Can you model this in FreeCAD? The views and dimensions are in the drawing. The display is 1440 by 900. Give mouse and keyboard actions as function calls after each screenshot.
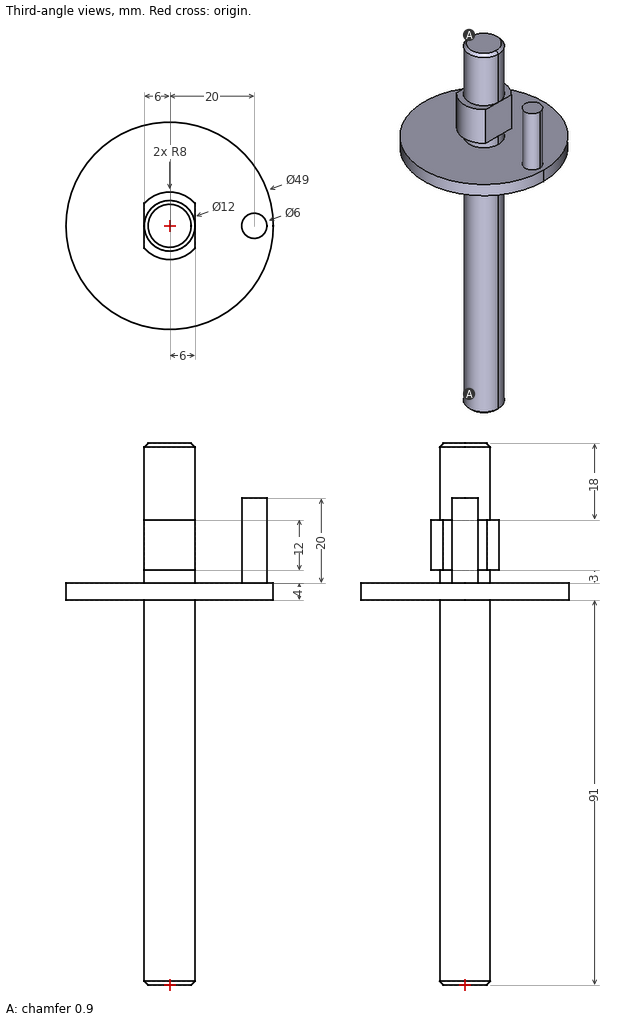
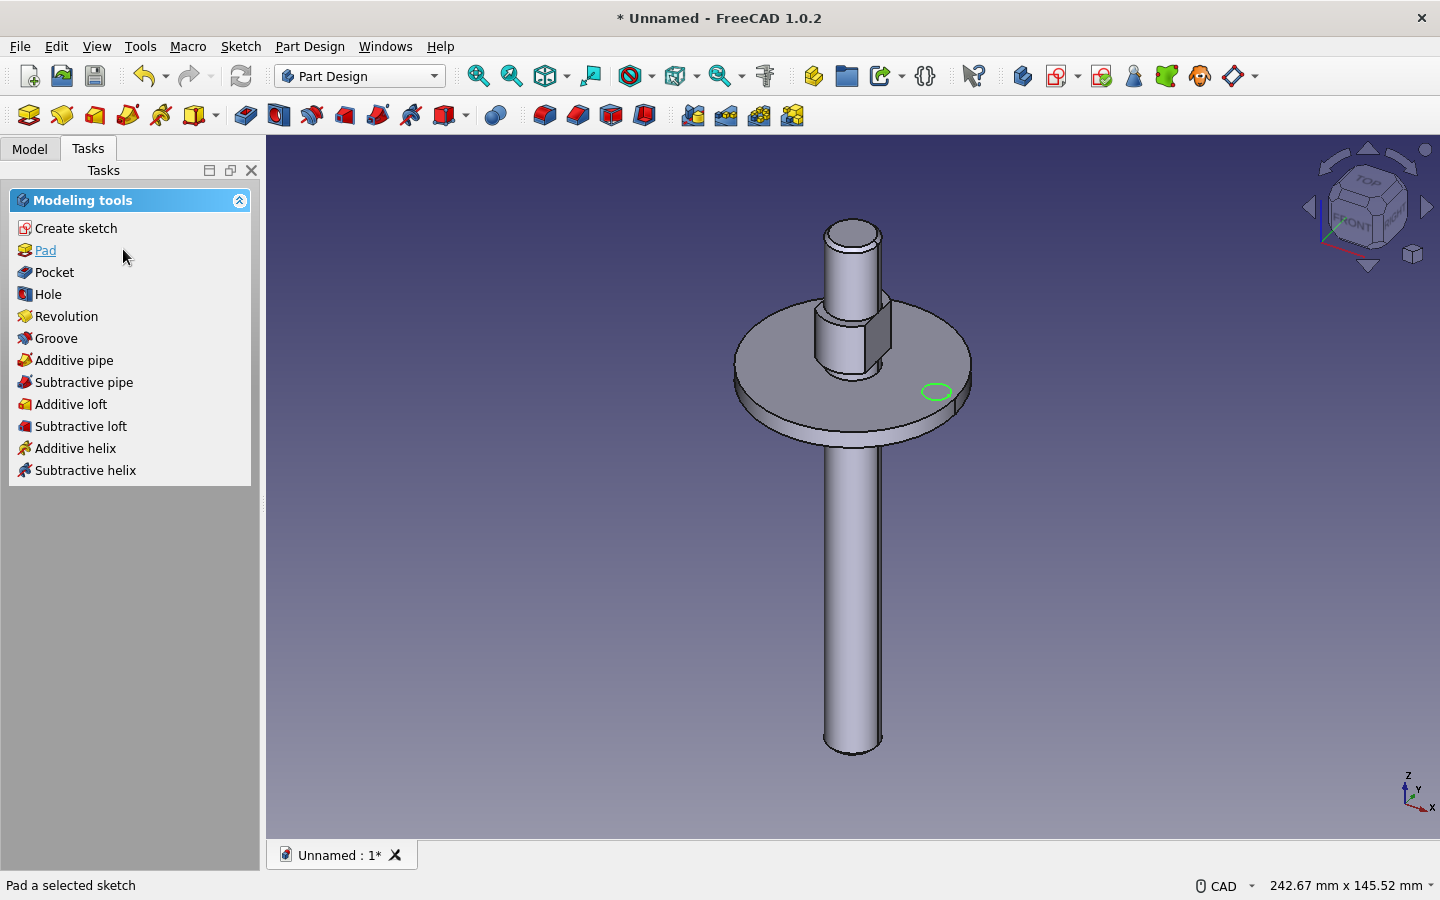
click(29, 116)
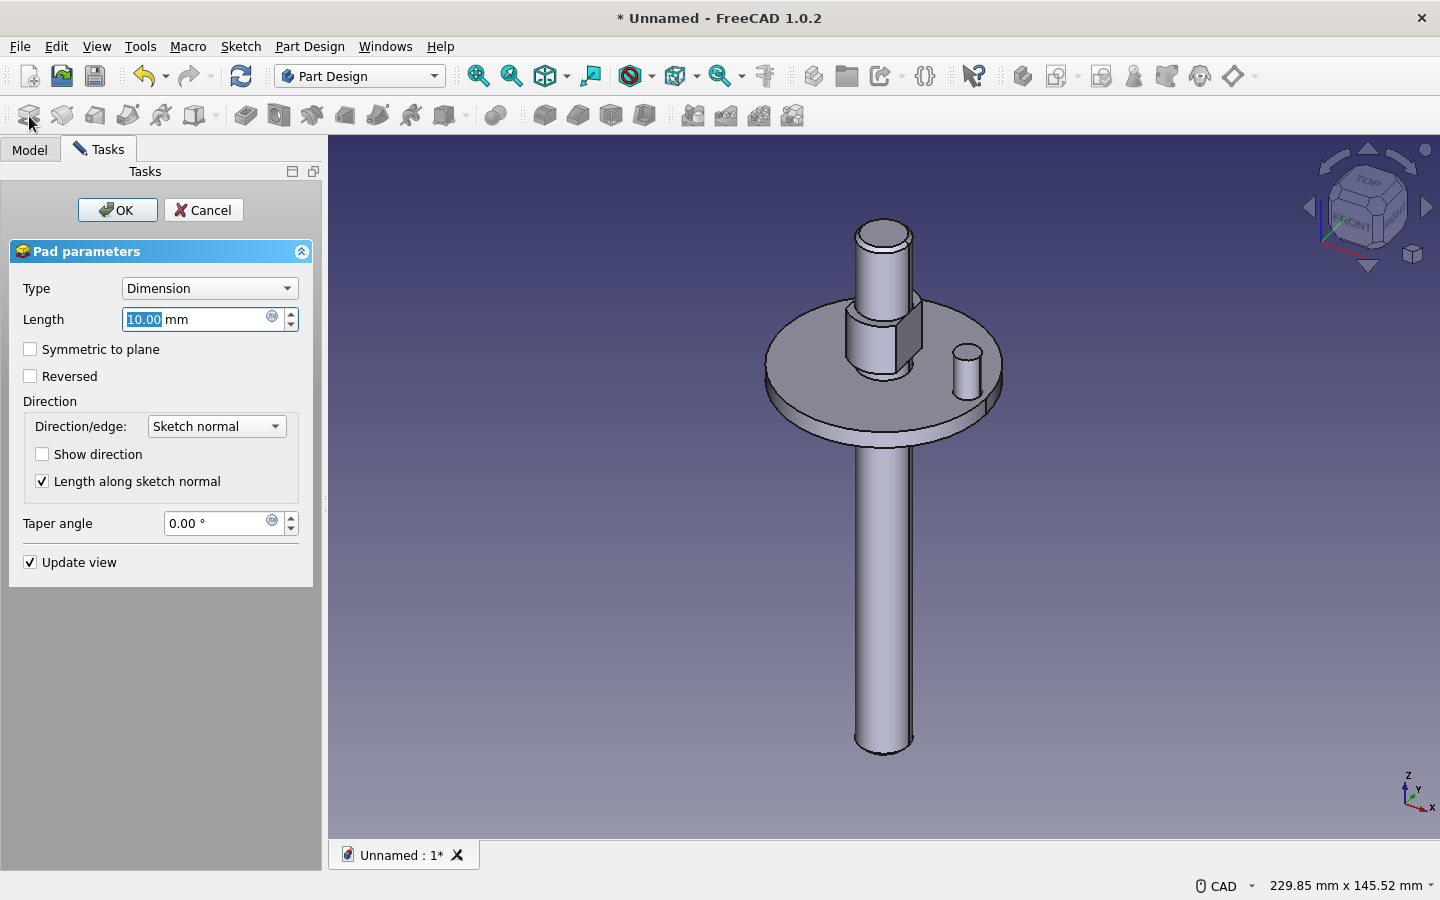
text(20)
key(Tab)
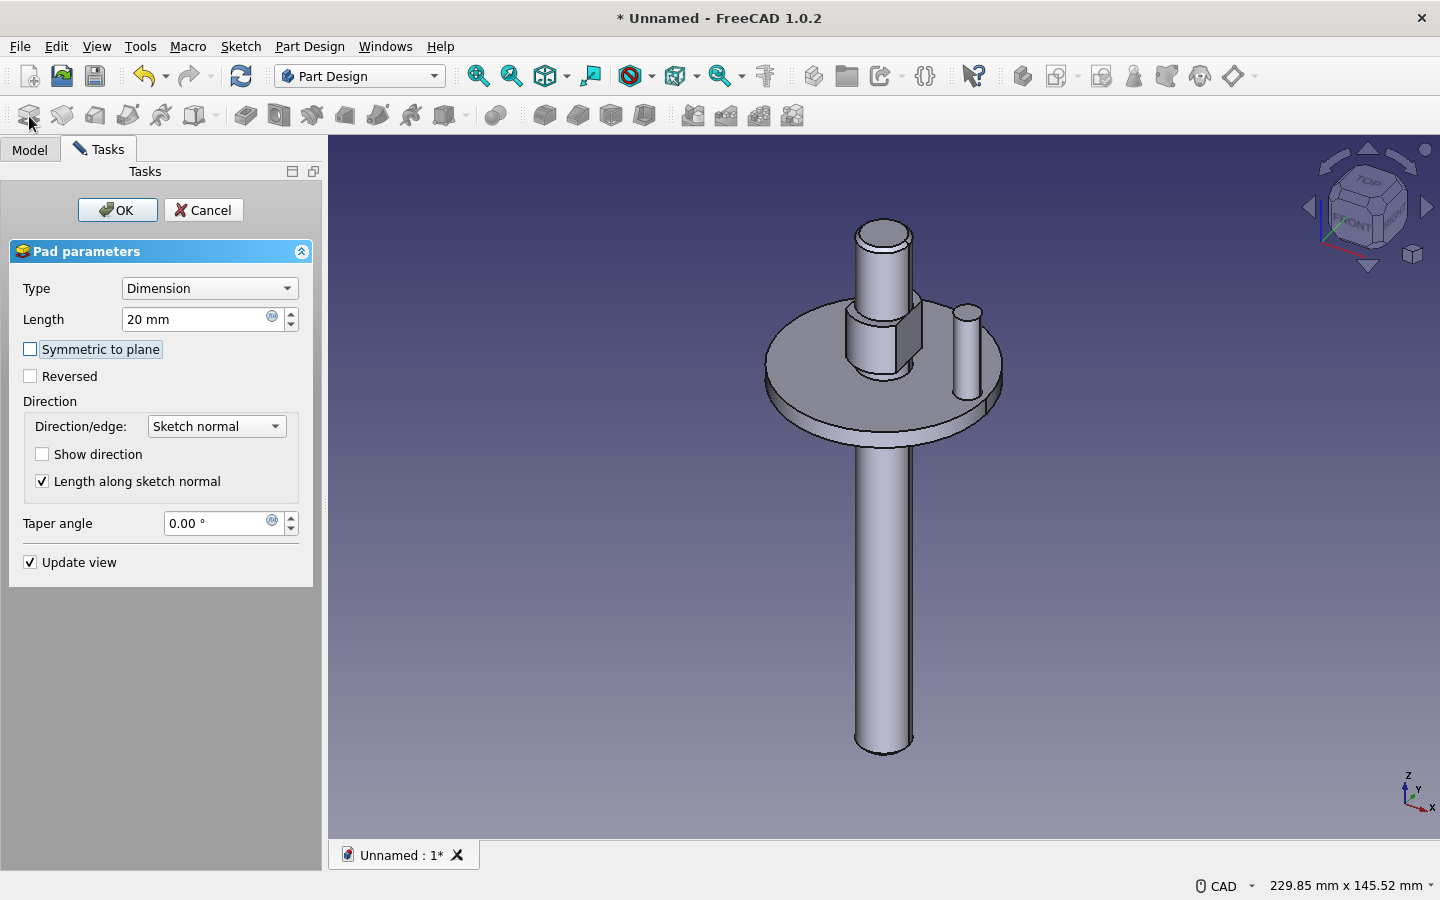
click(118, 210)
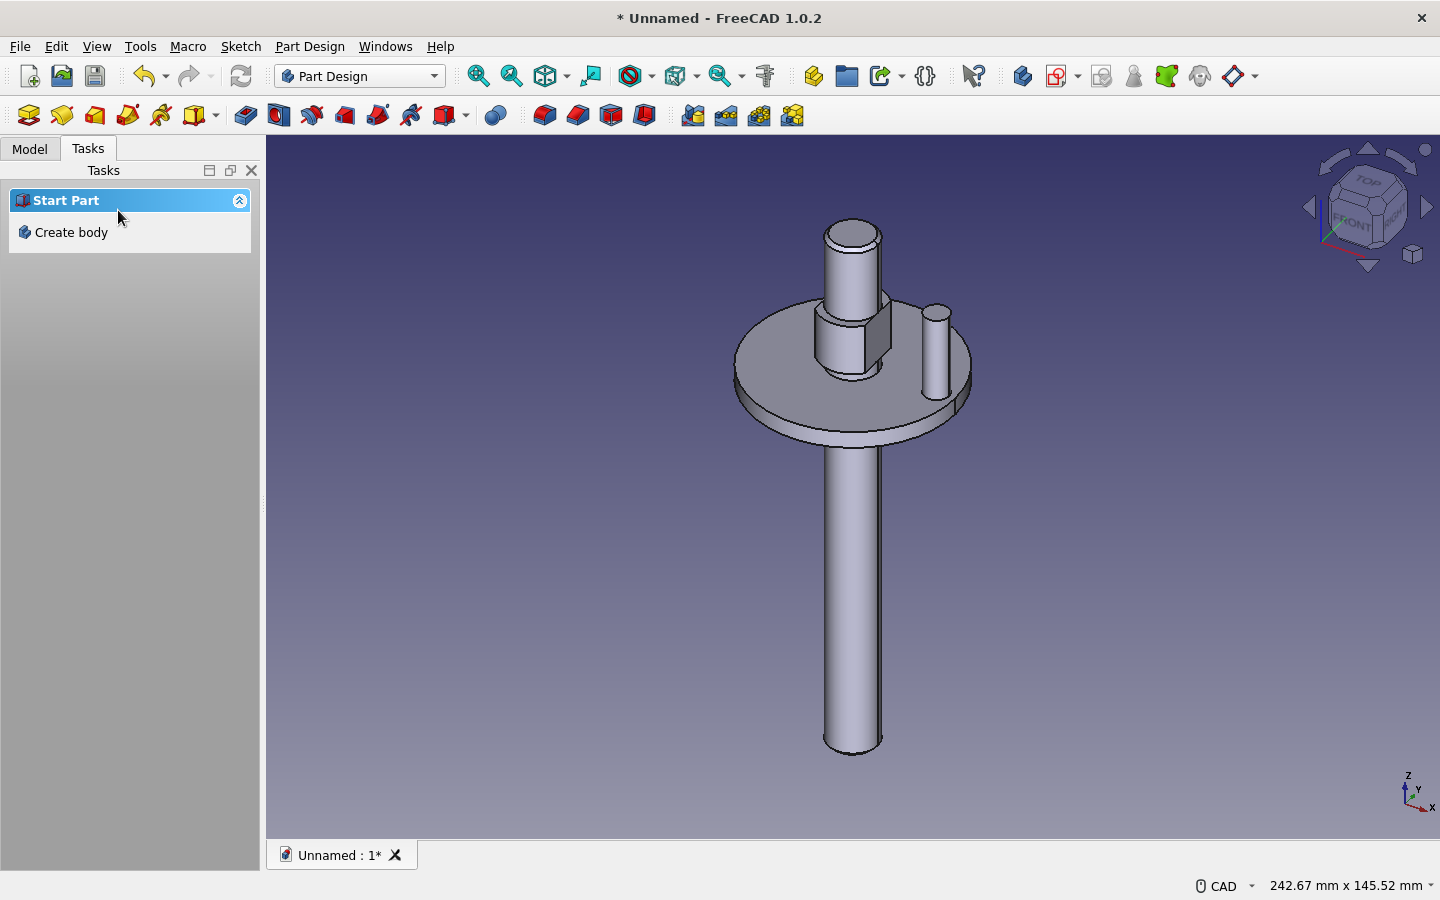
key(0)